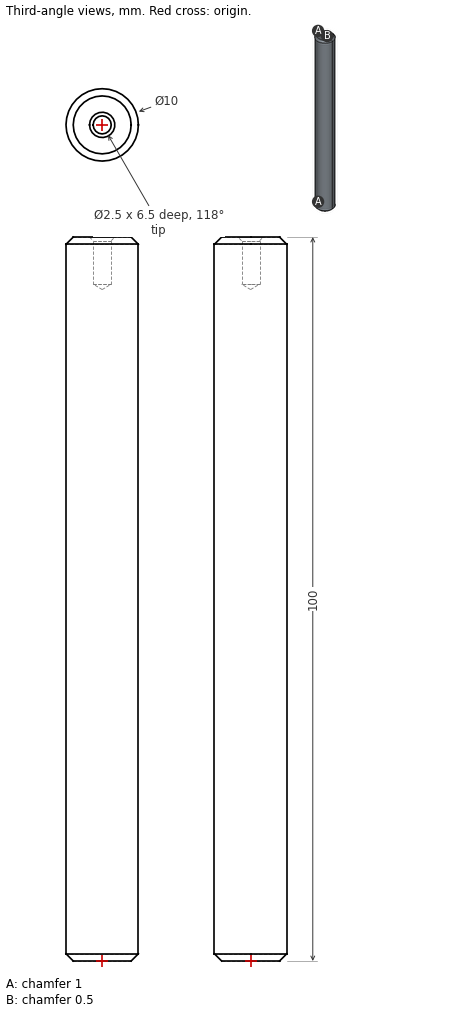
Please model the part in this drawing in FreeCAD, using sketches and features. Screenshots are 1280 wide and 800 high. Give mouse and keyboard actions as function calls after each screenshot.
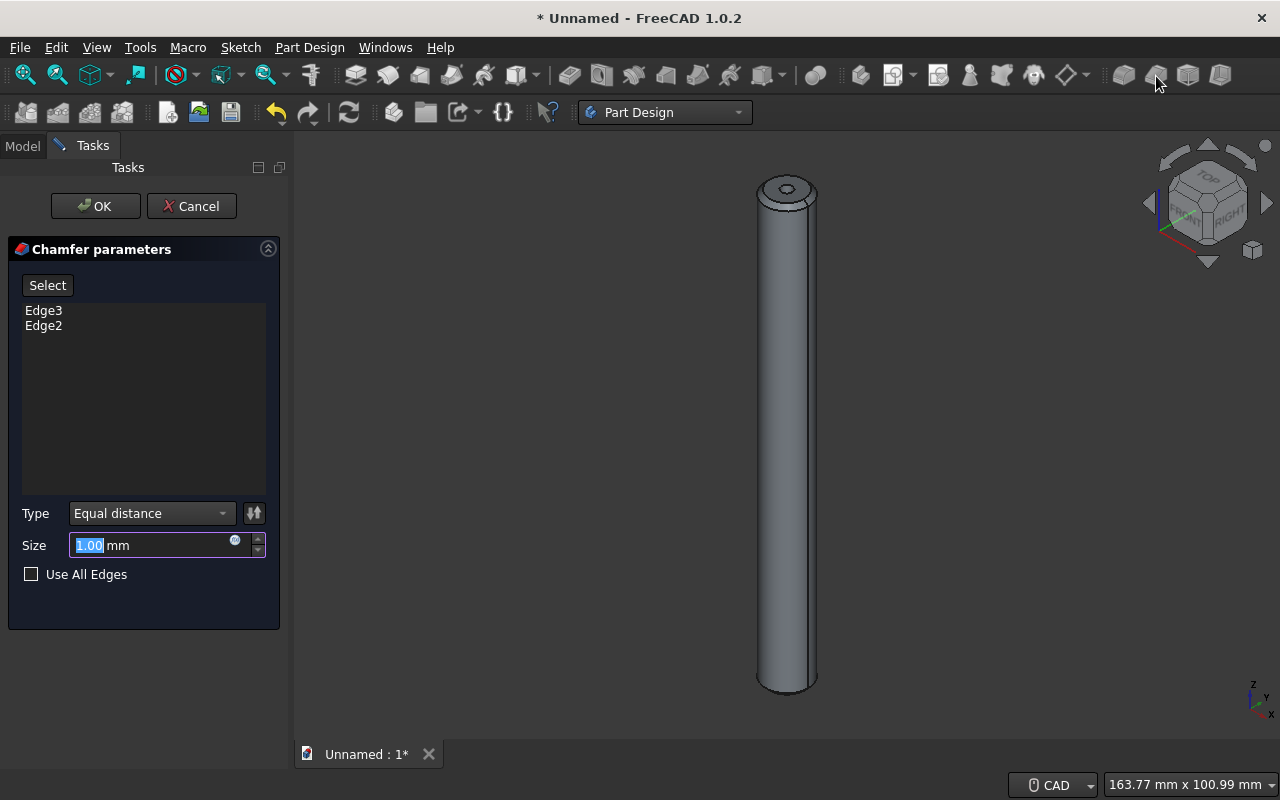
text(1)
key(Tab)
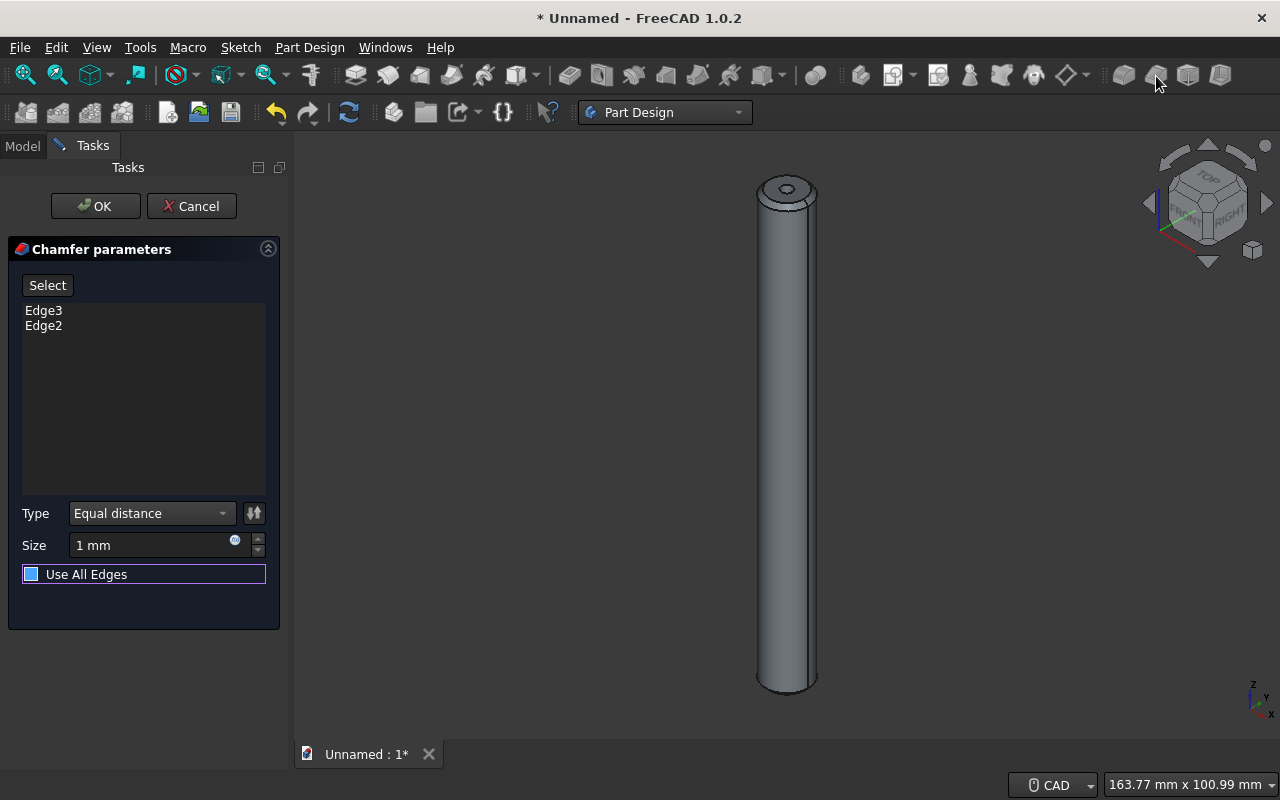
click(96, 206)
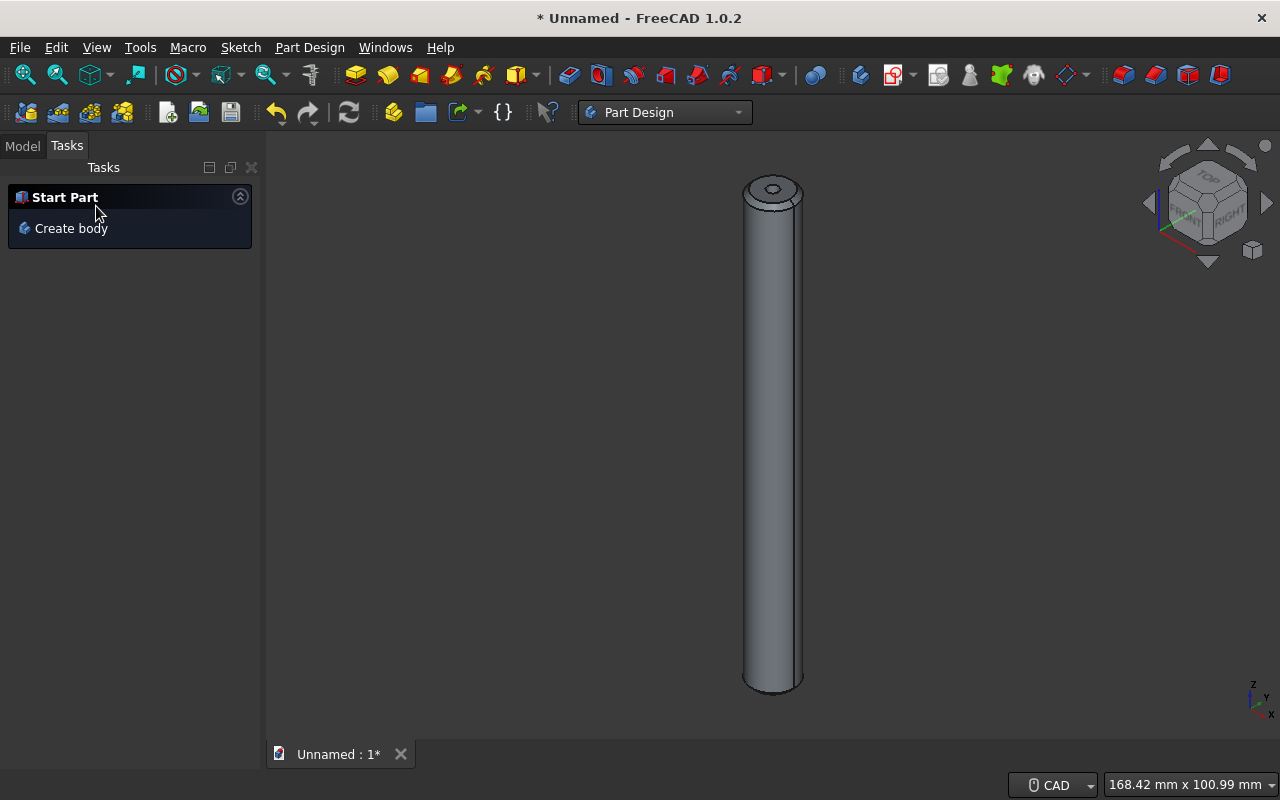
click(768, 185)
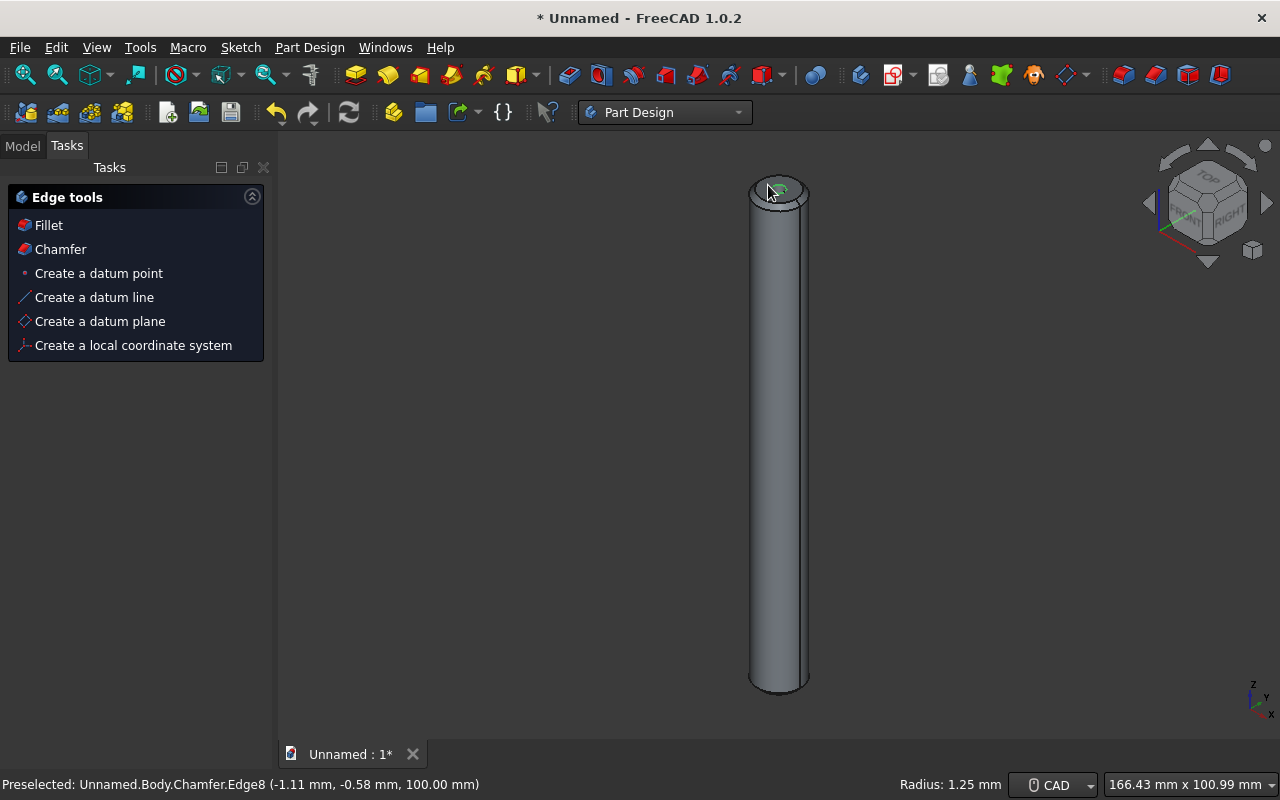
click(1156, 76)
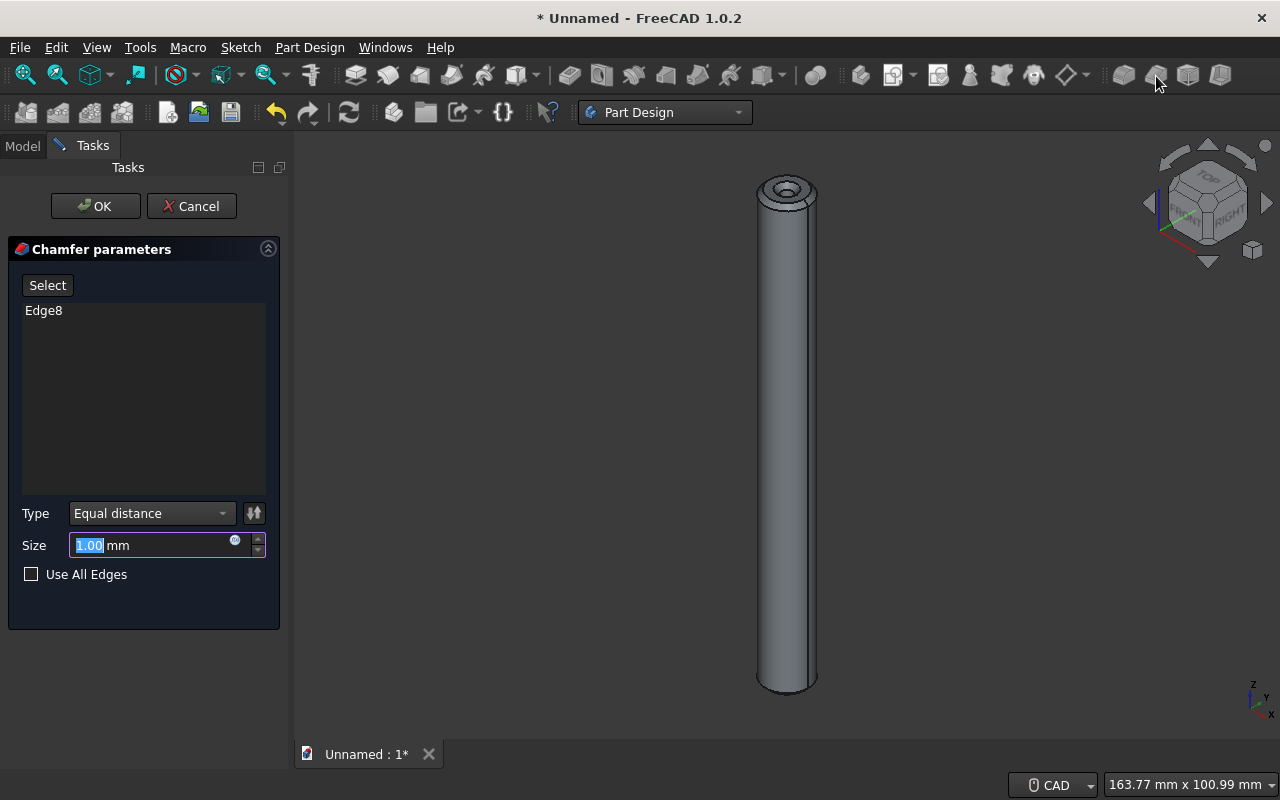
text(0.5)
key(Tab)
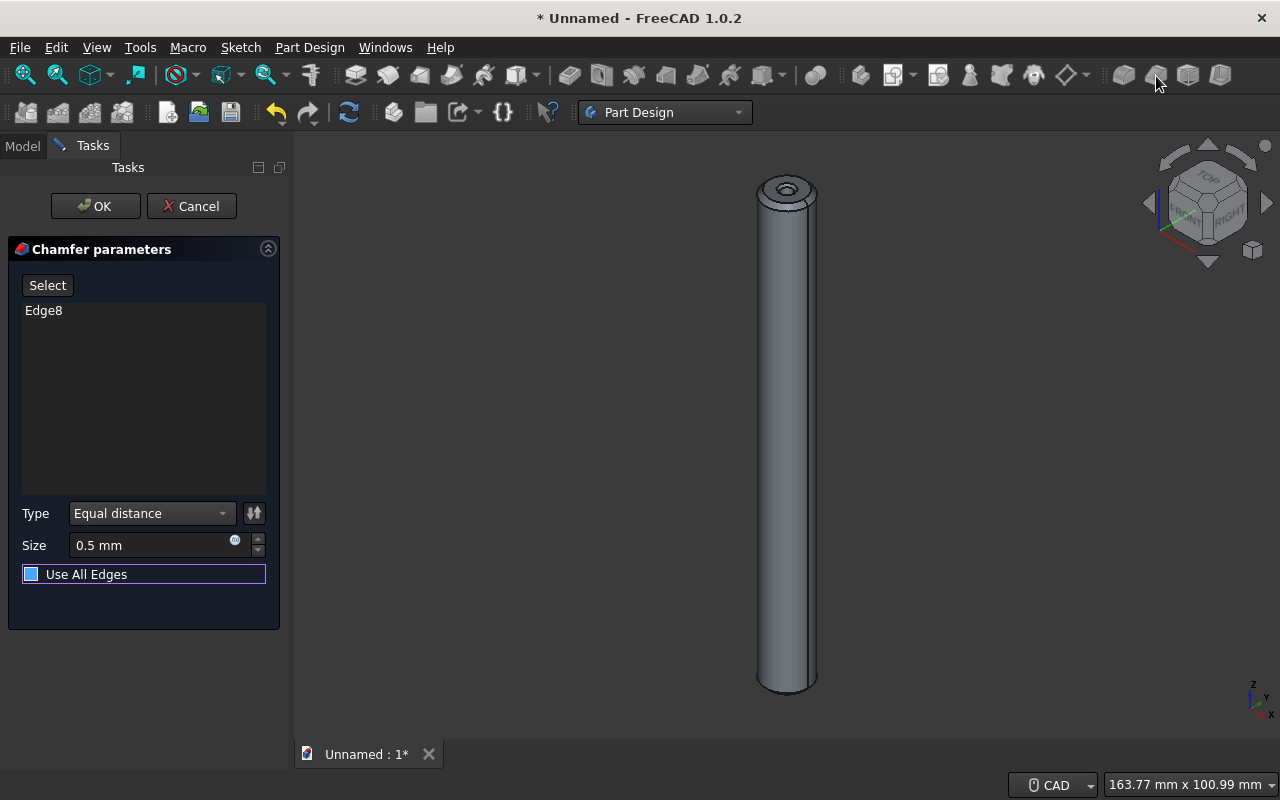
click(96, 206)